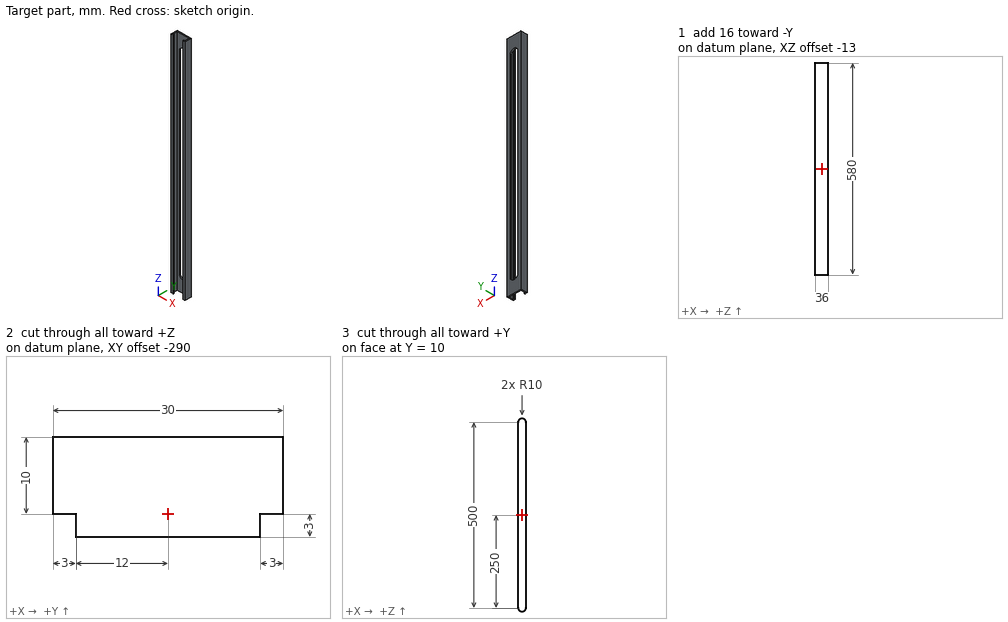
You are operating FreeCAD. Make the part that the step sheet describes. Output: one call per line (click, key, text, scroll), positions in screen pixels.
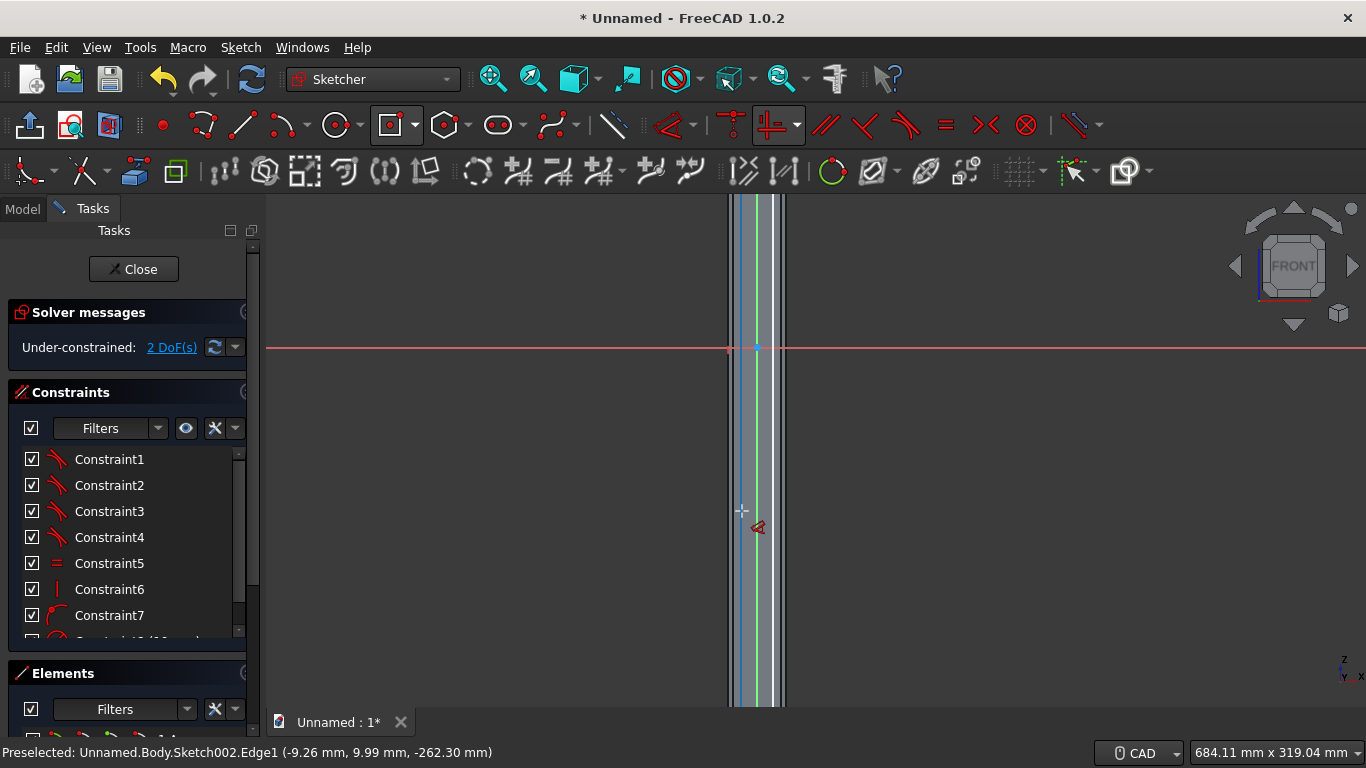
click(741, 510)
click(707, 450)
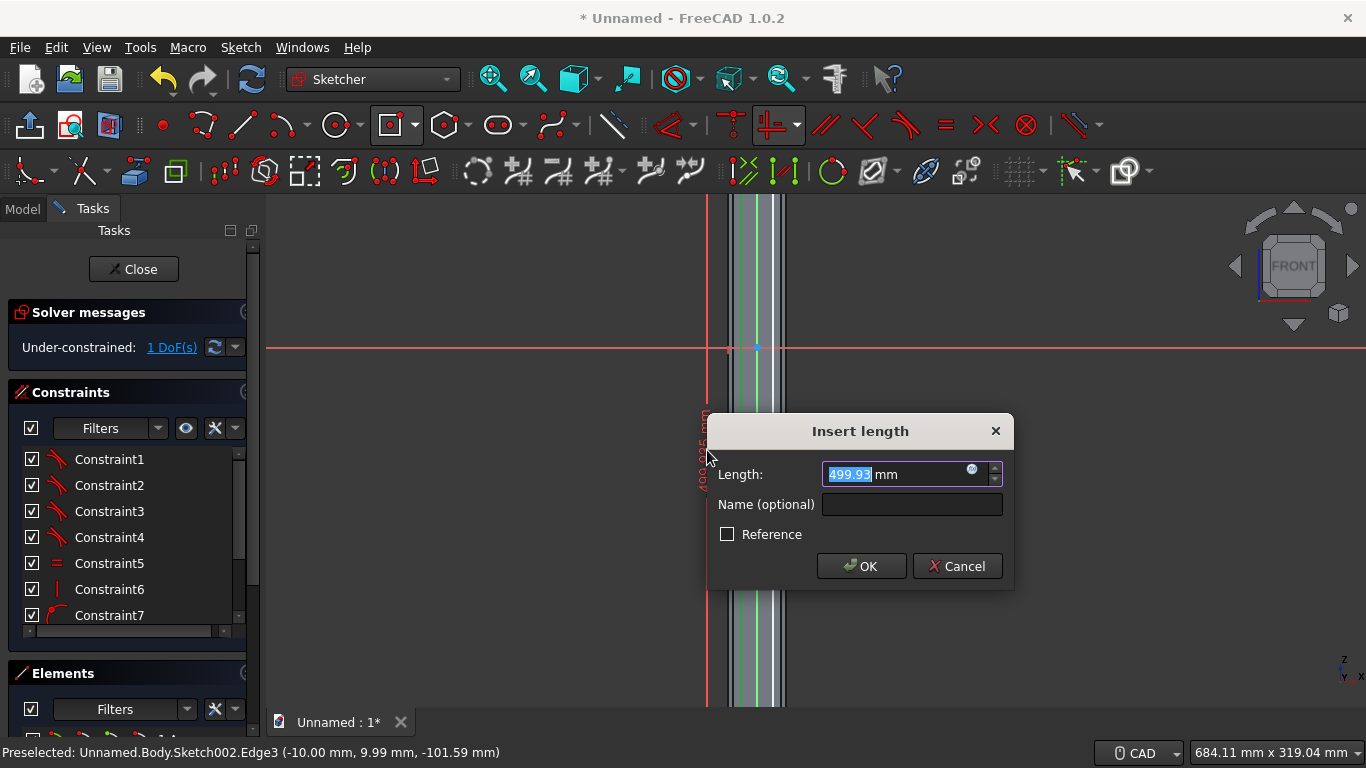
text(500)
key(Return)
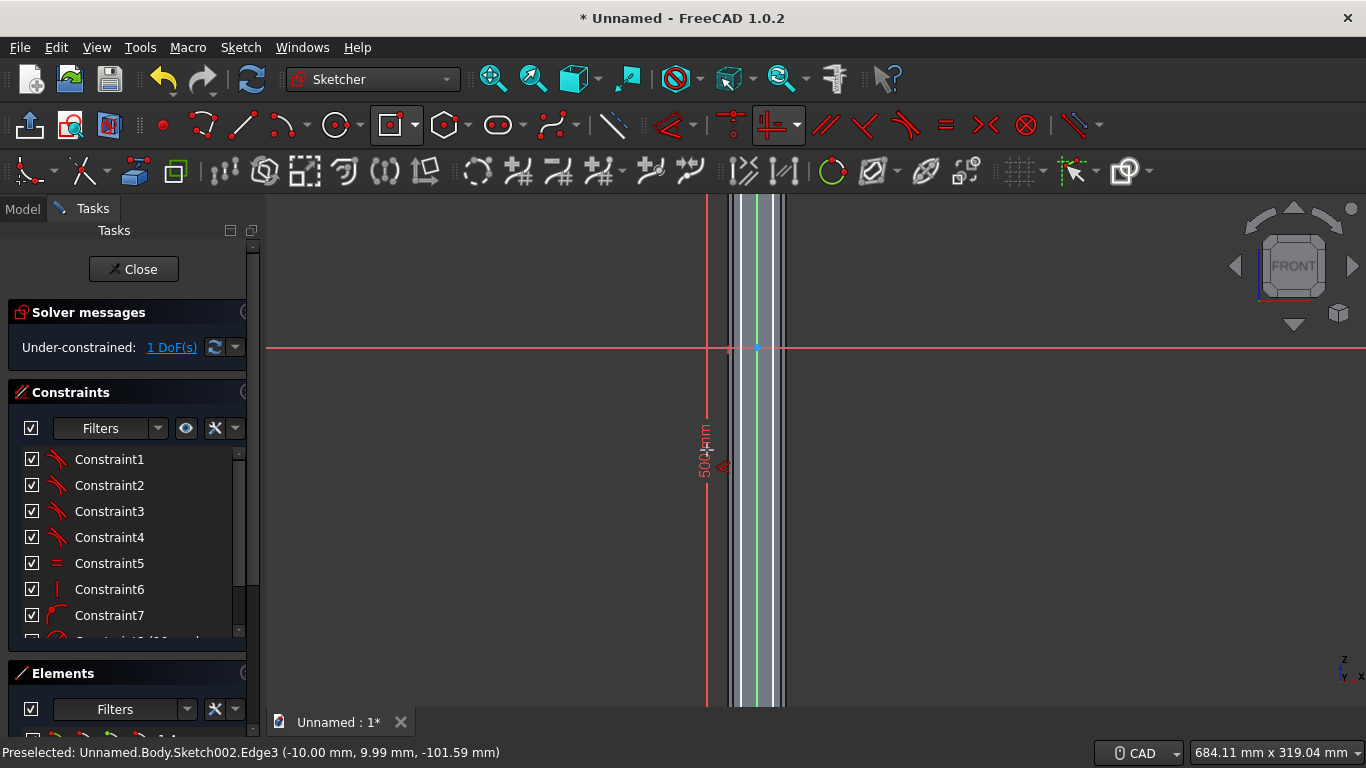
scroll(742, 510, down, 5)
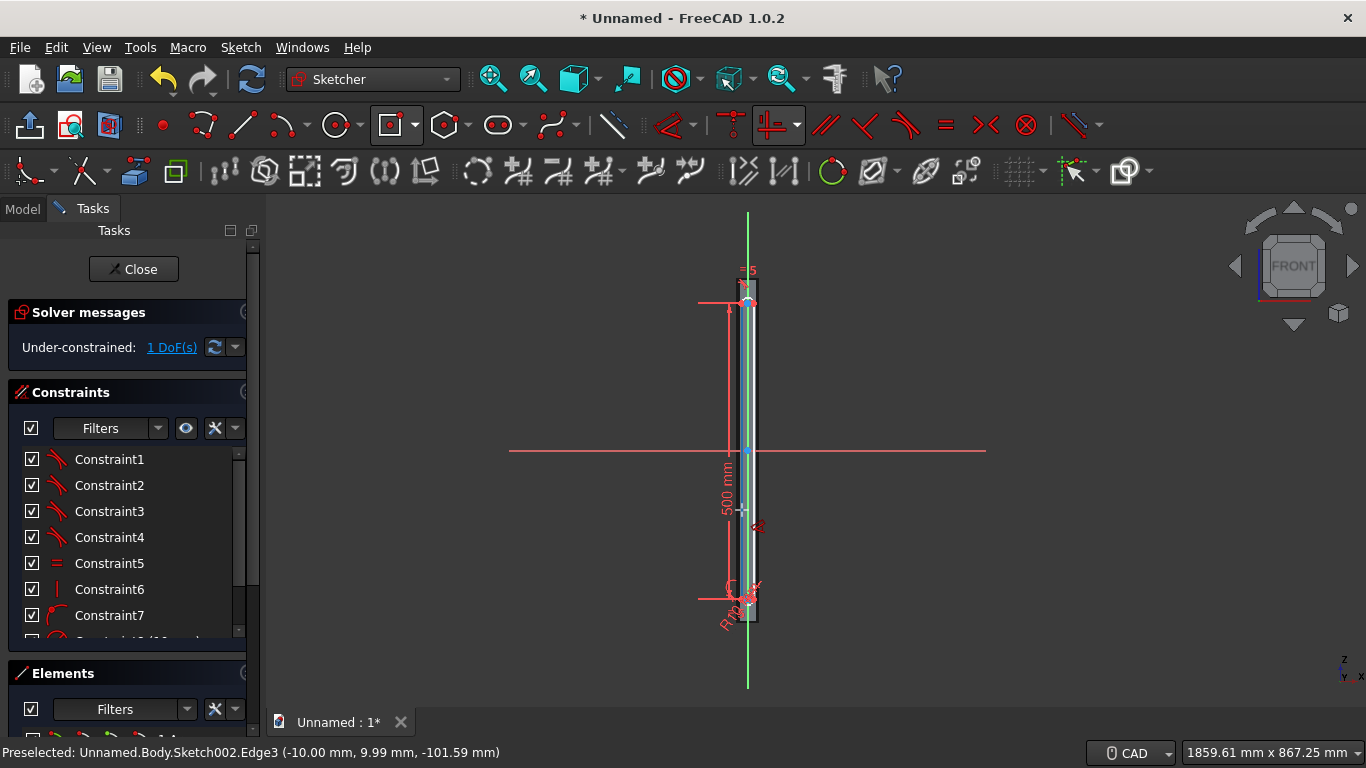
scroll(742, 599, up, 4)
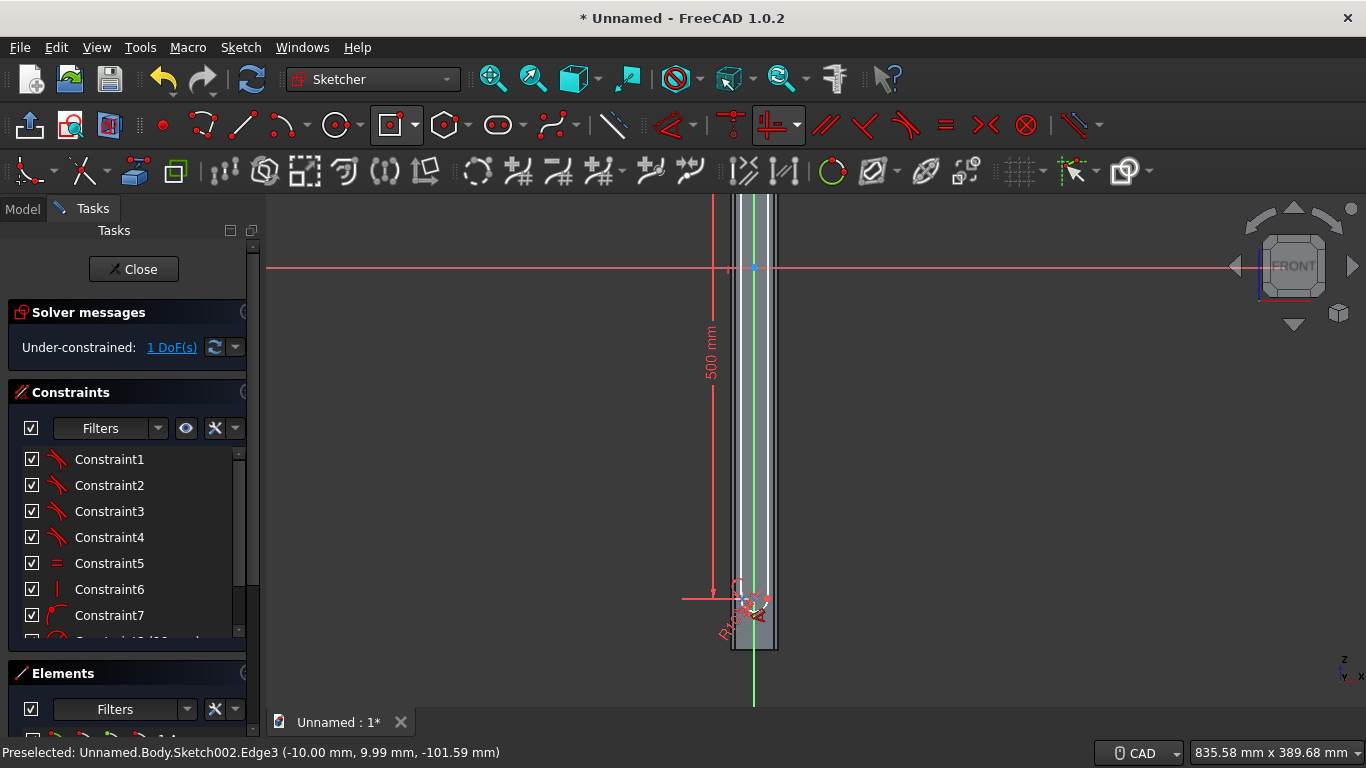
click(741, 599)
click(707, 433)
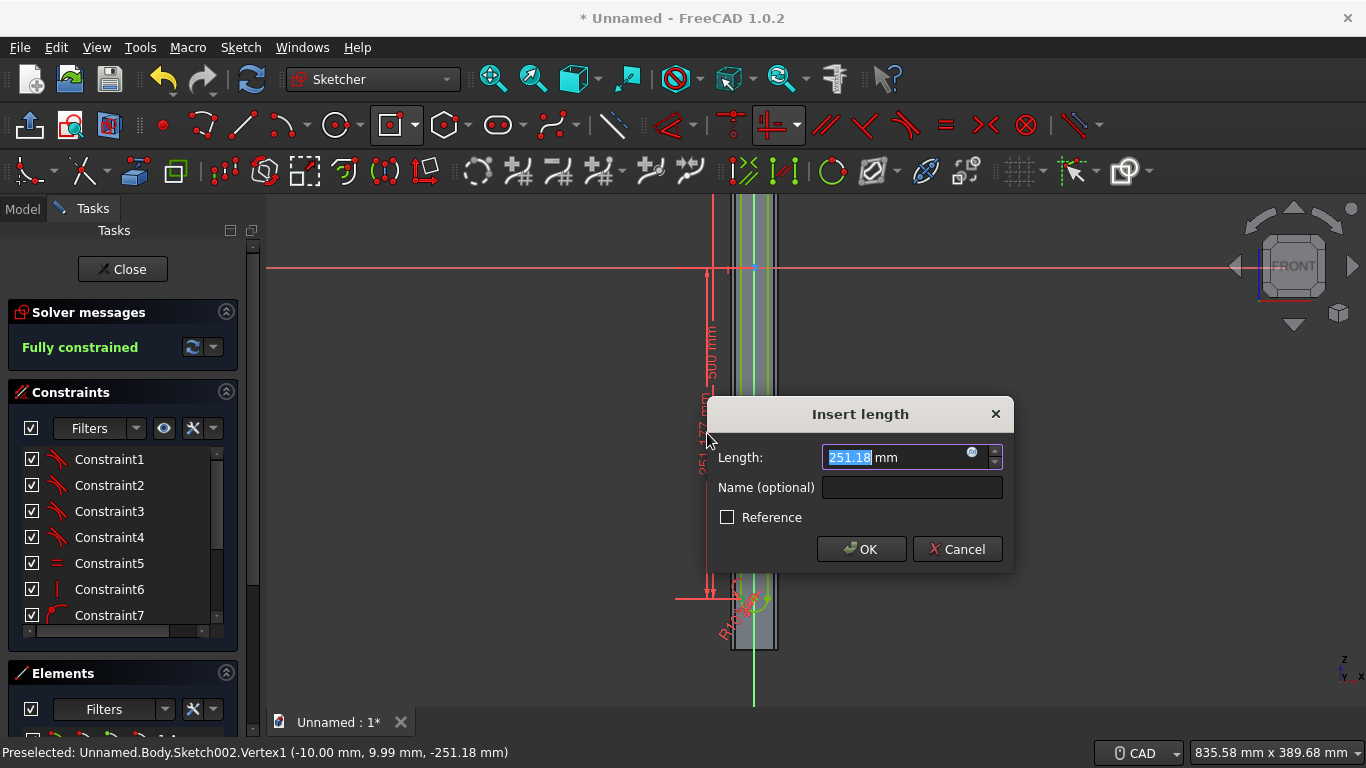
text(250)
key(Return)
key(Escape)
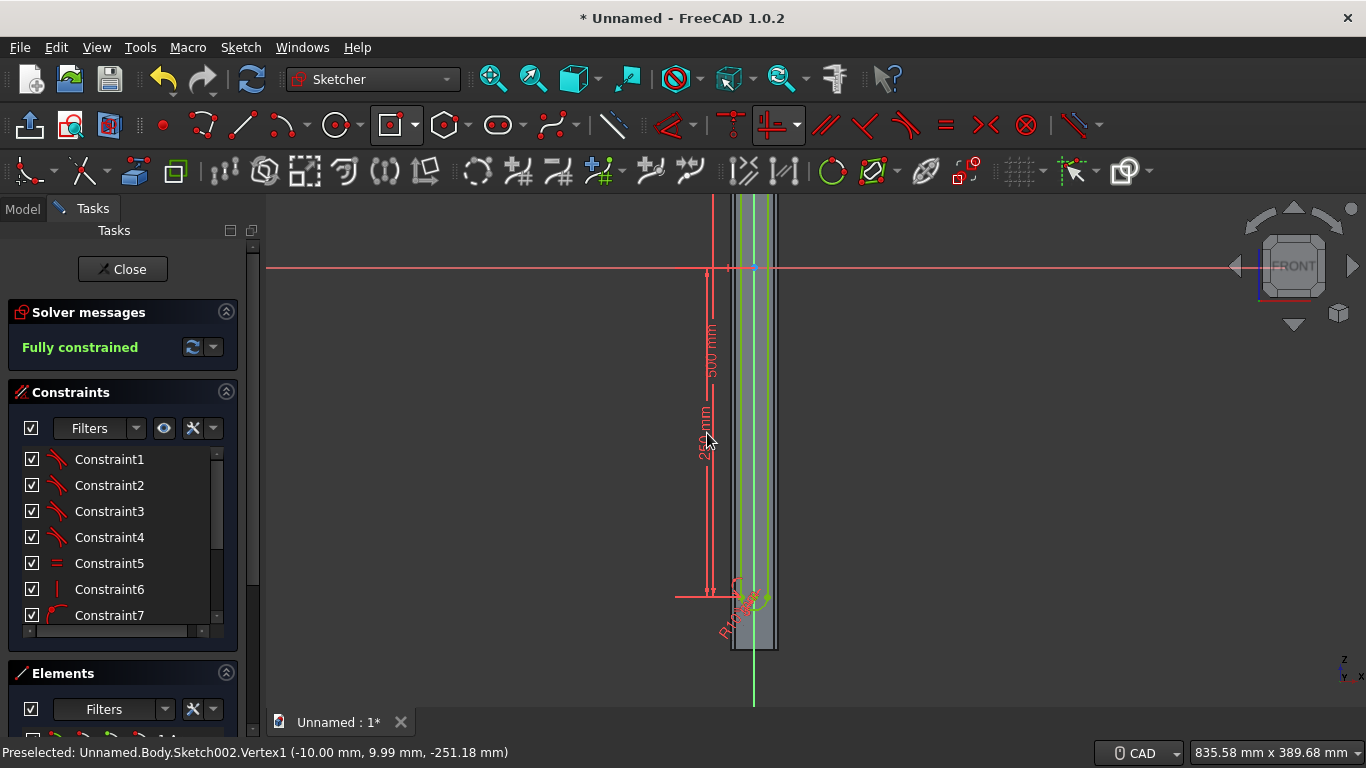
click(123, 269)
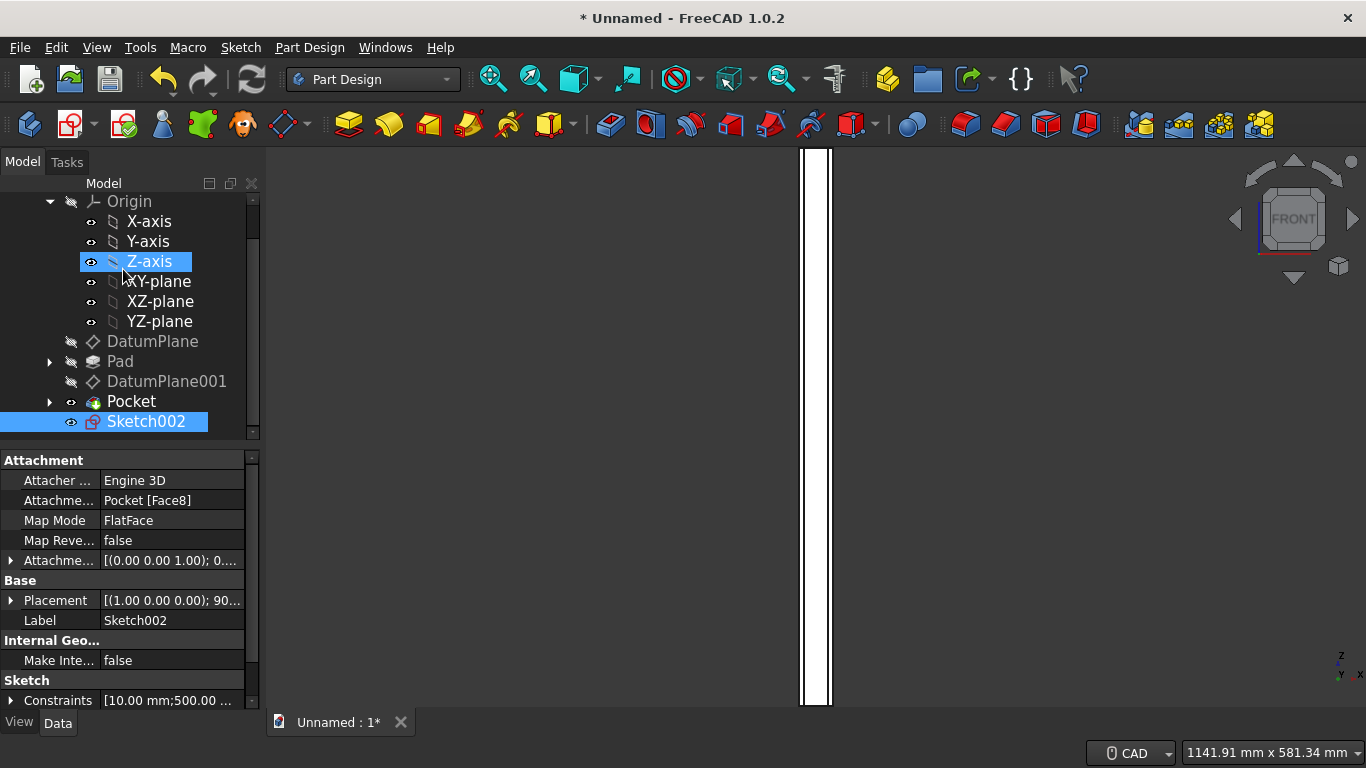
click(612, 124)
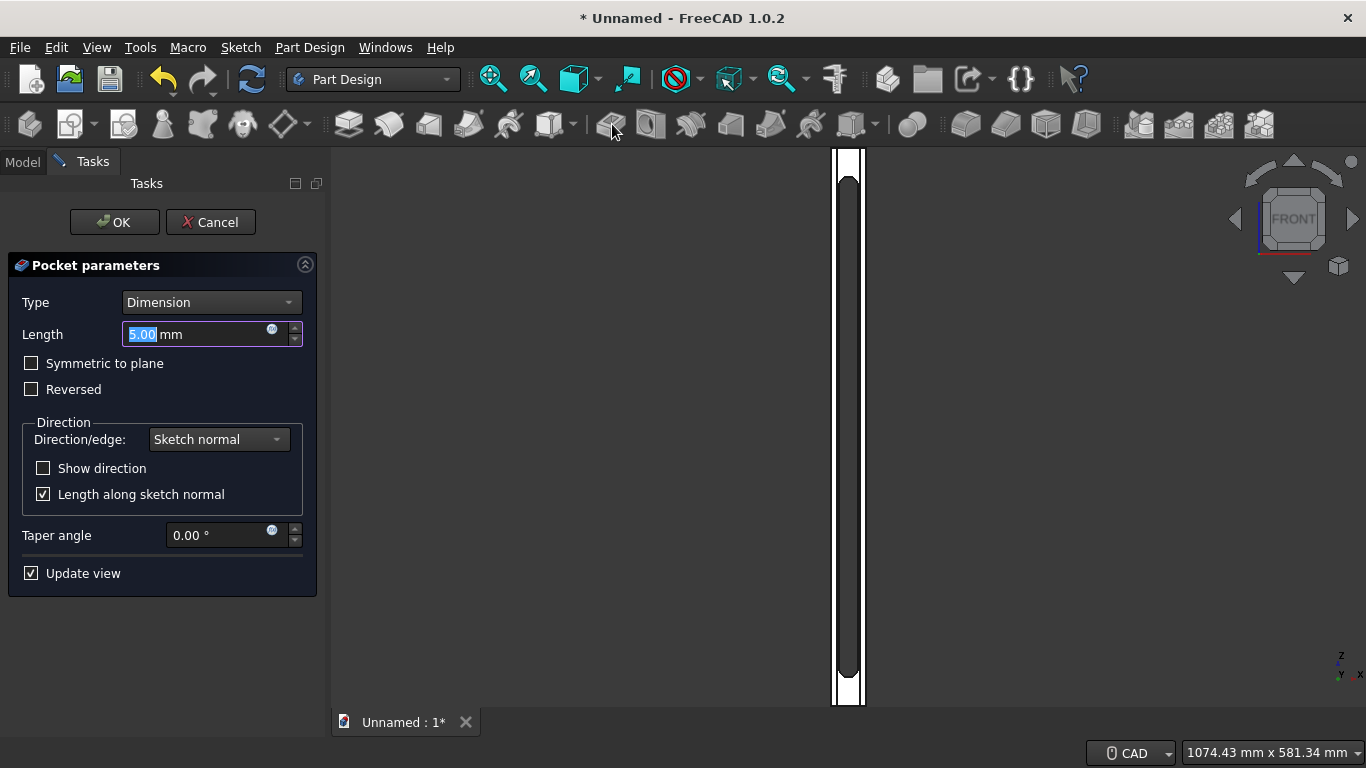
click(212, 302)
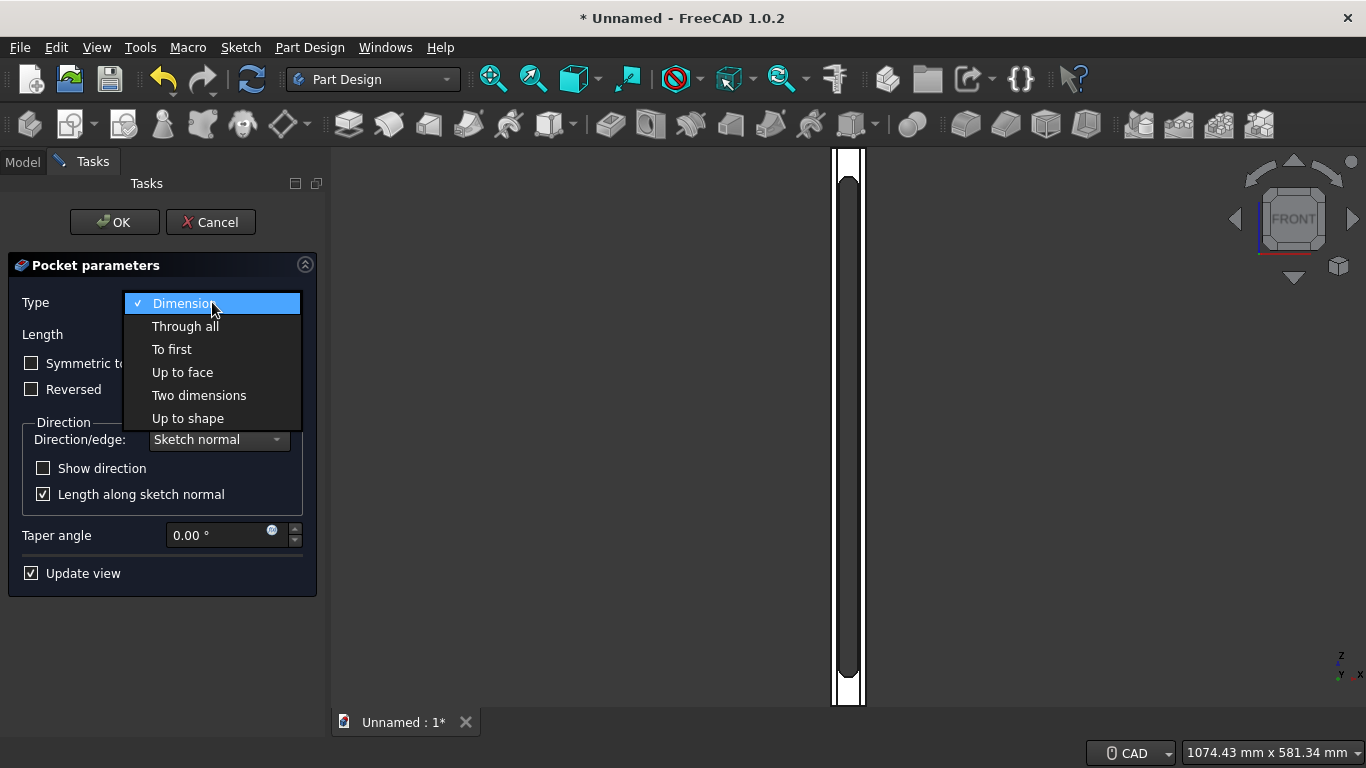
click(212, 326)